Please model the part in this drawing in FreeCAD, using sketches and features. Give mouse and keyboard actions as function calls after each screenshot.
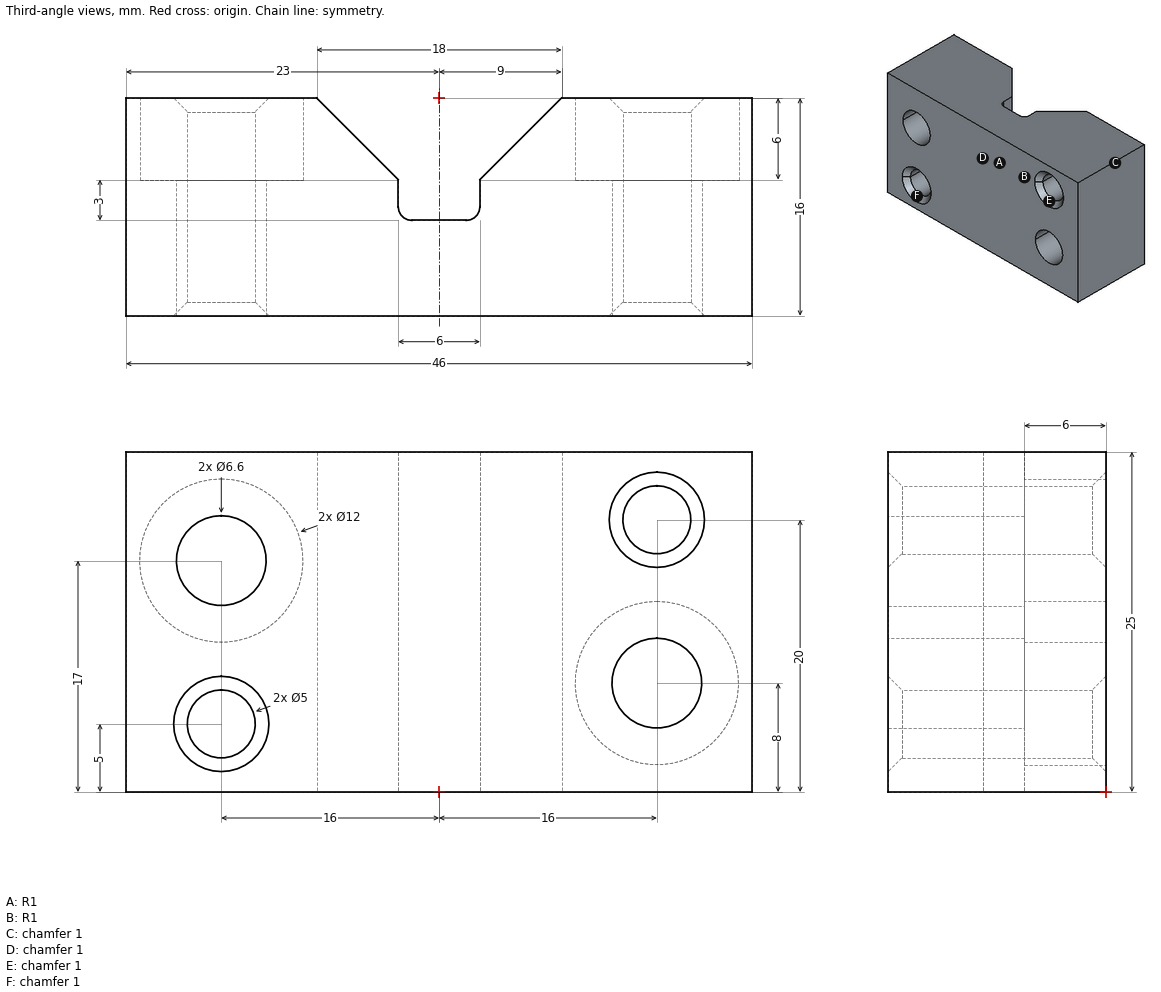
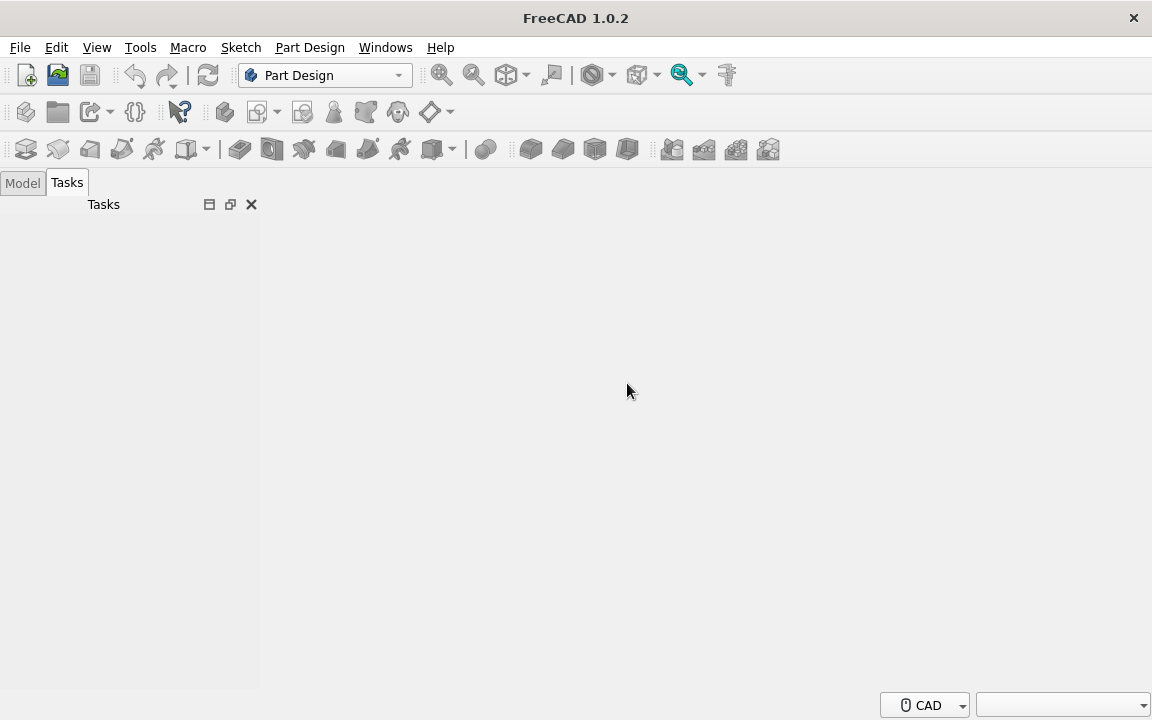
click(26, 76)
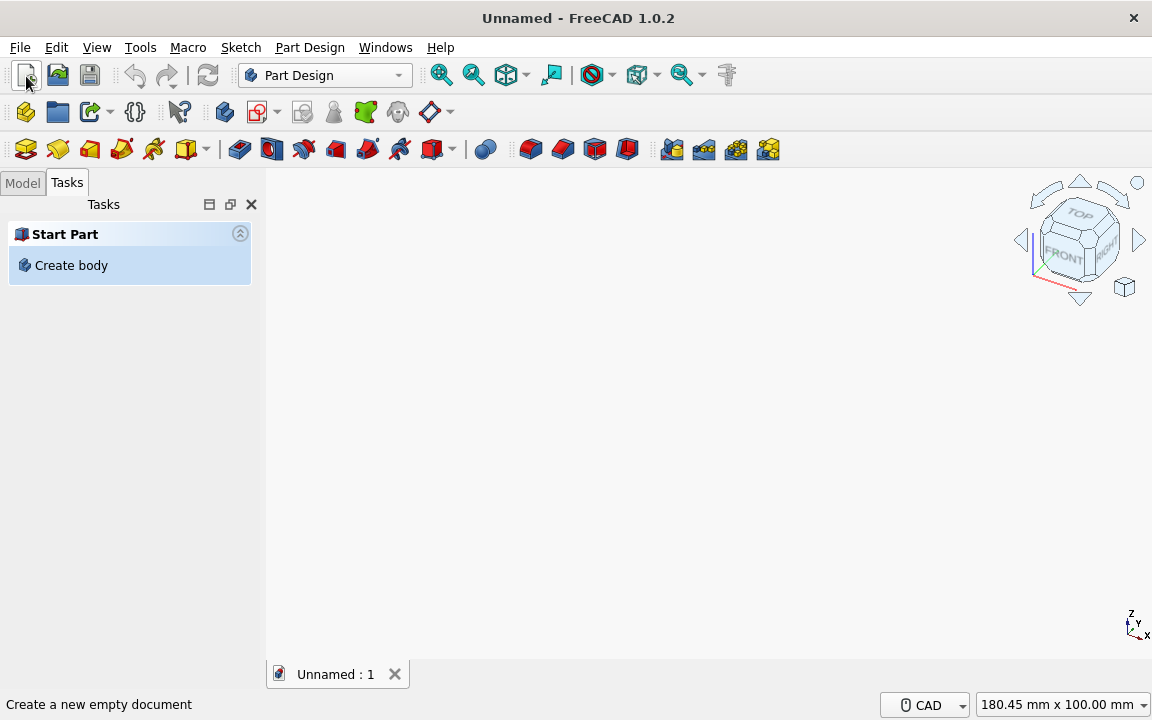
click(258, 112)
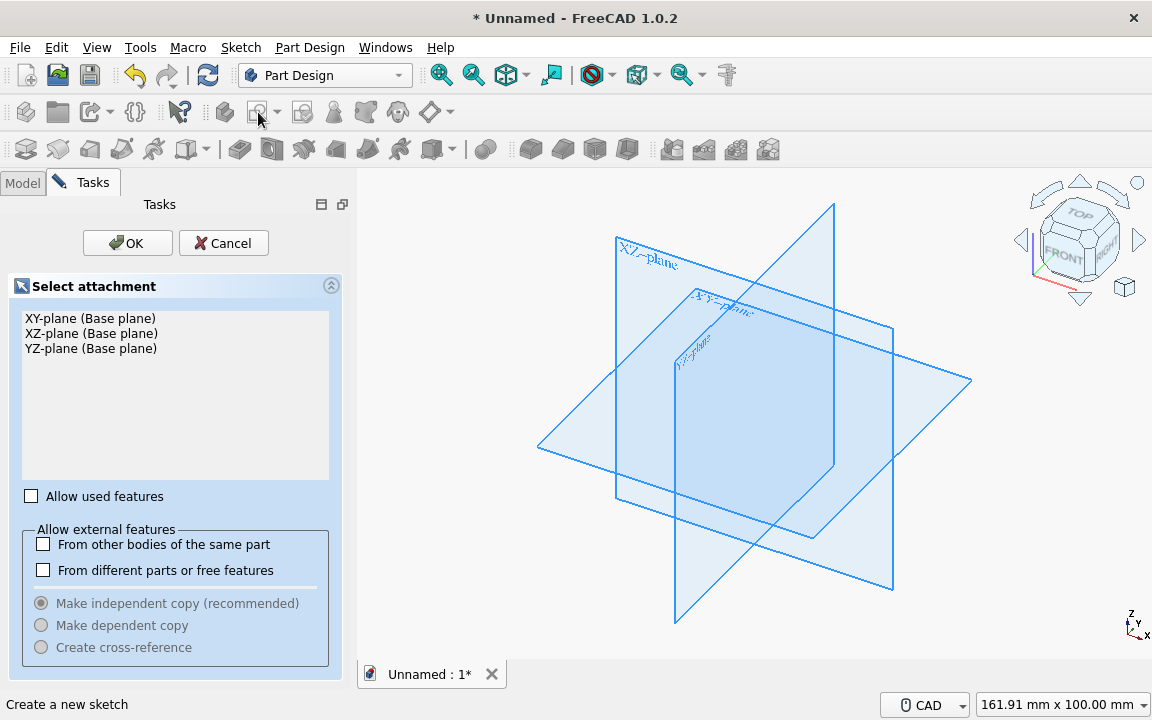
click(82, 318)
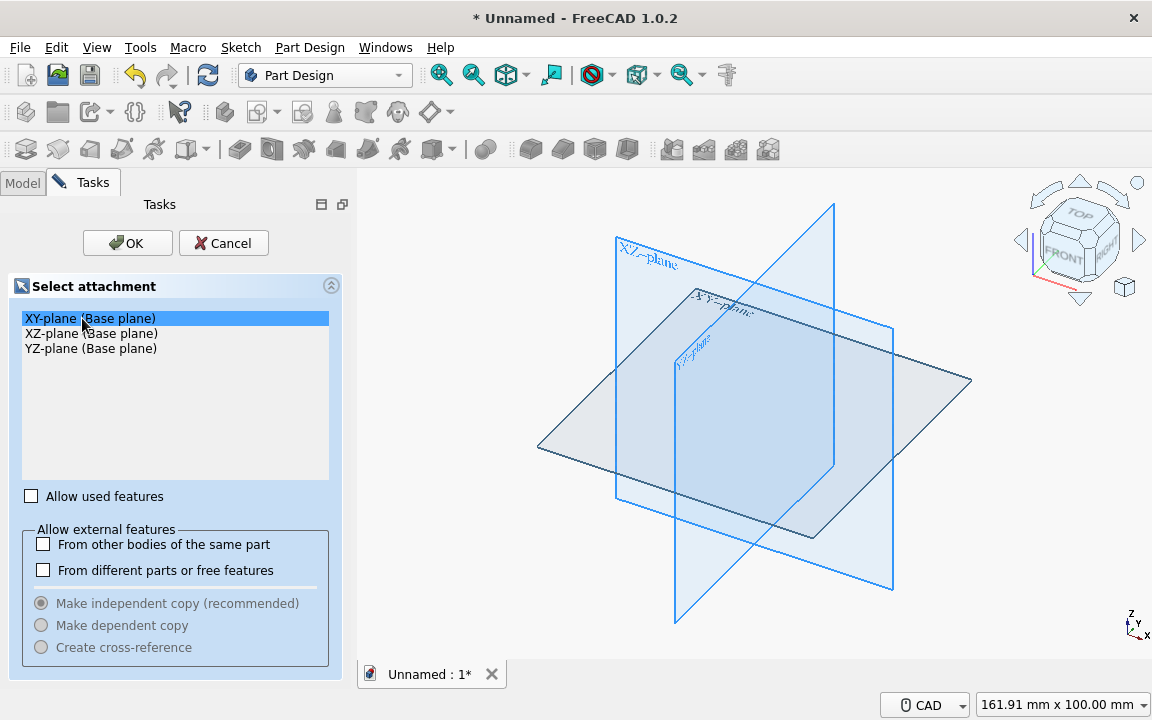
click(128, 243)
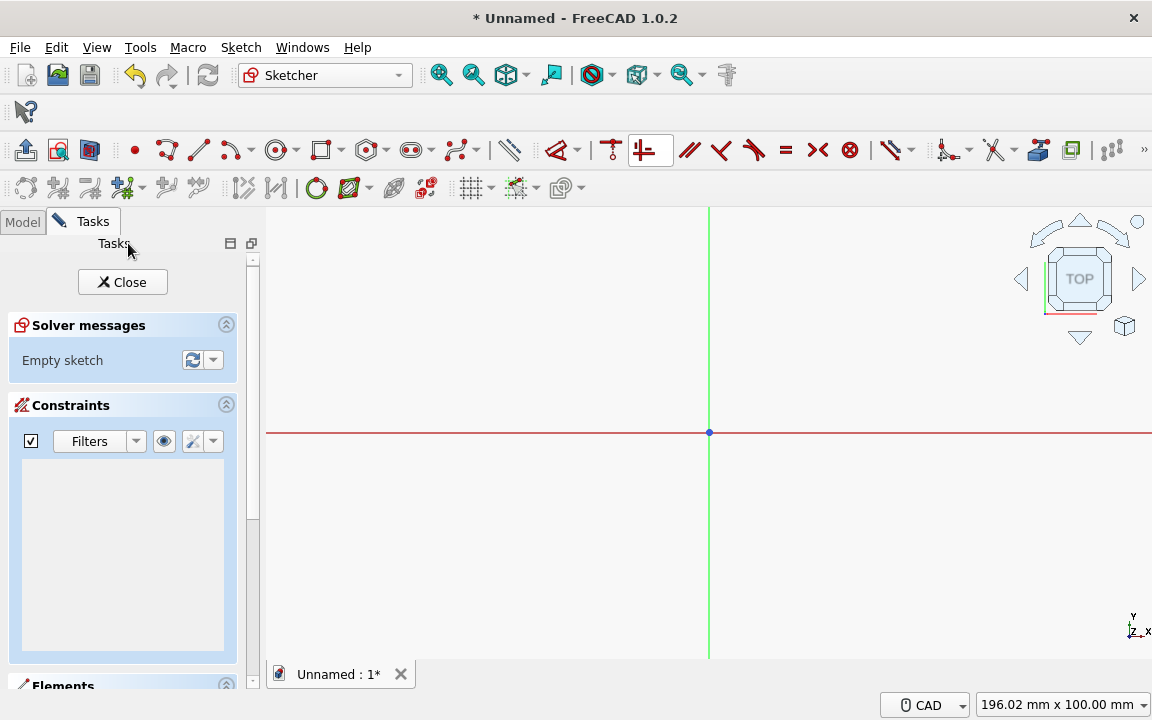
scroll(765, 499, up, 4)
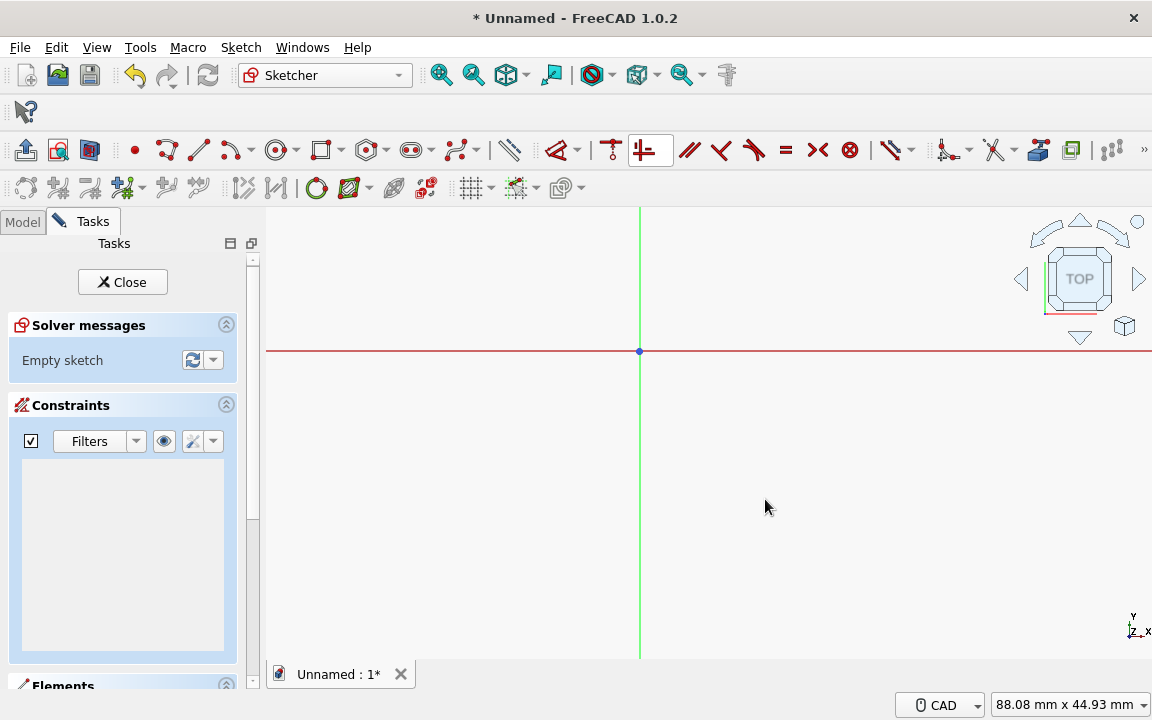
click(322, 150)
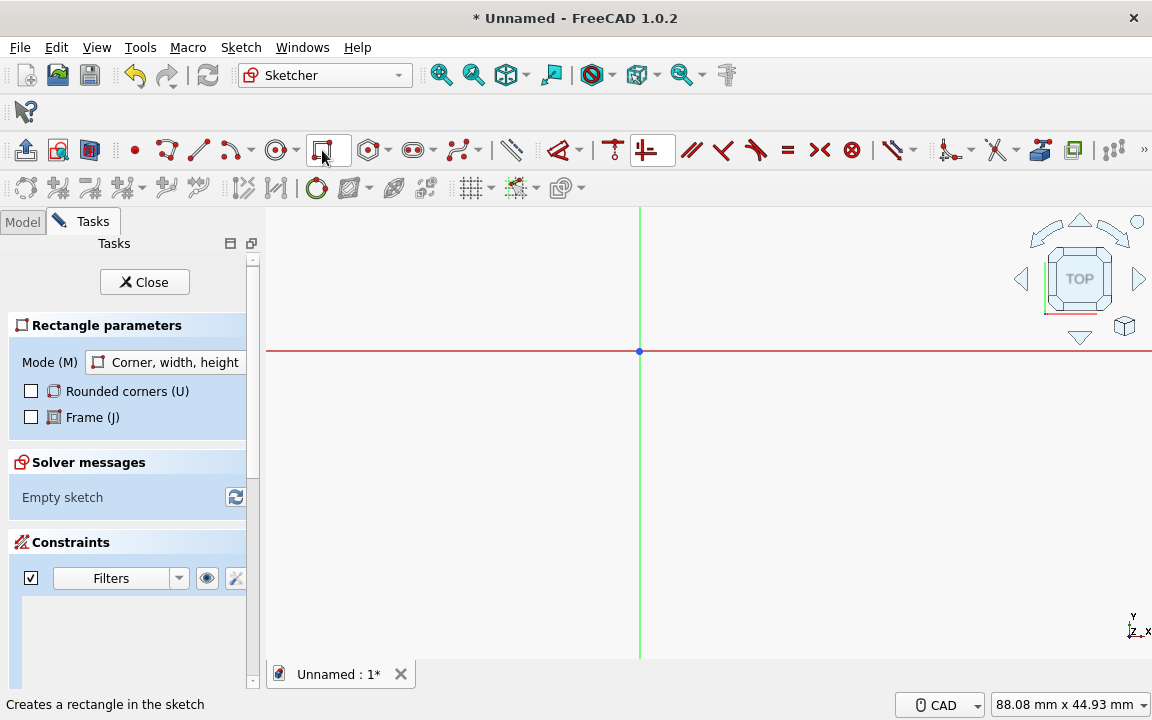
click(408, 351)
move(871, 512)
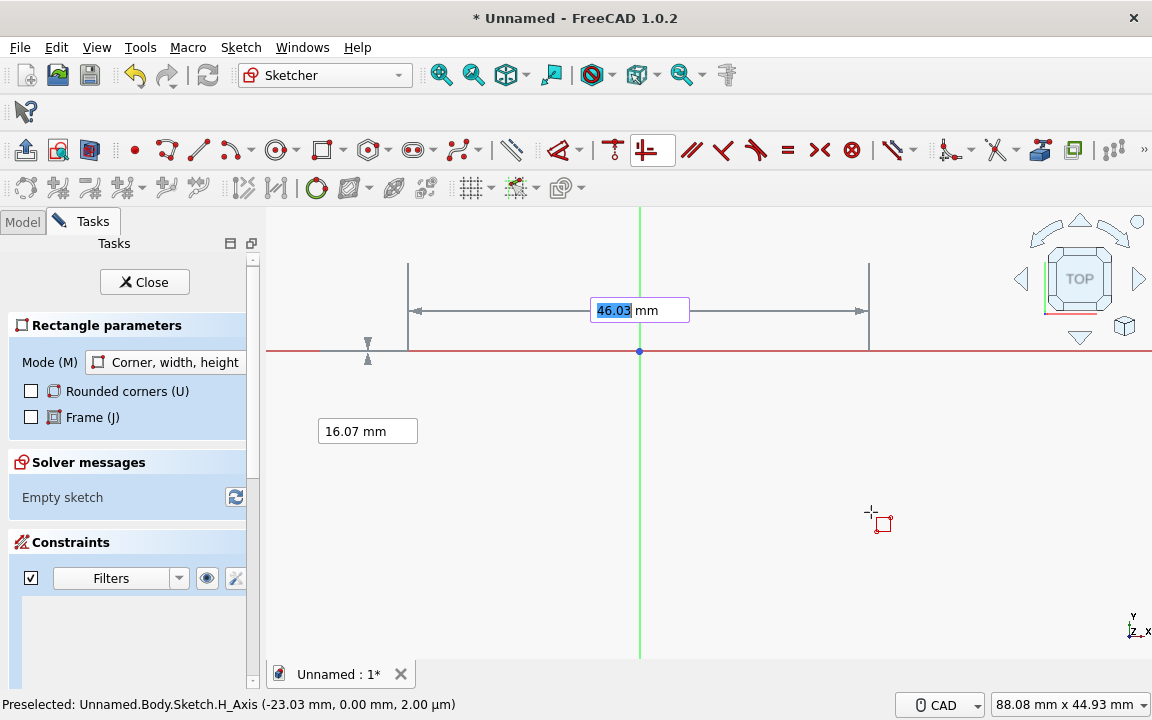
text(46)
key(Tab)
text(16)
key(Return)
key(Escape)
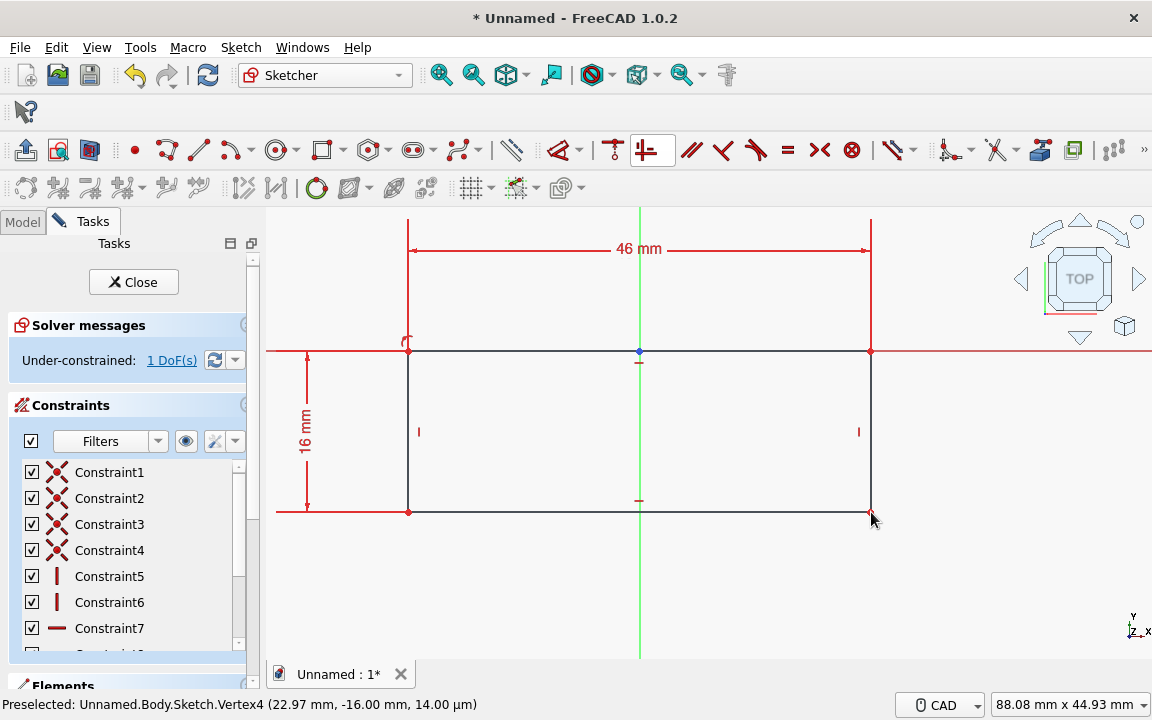
click(408, 351)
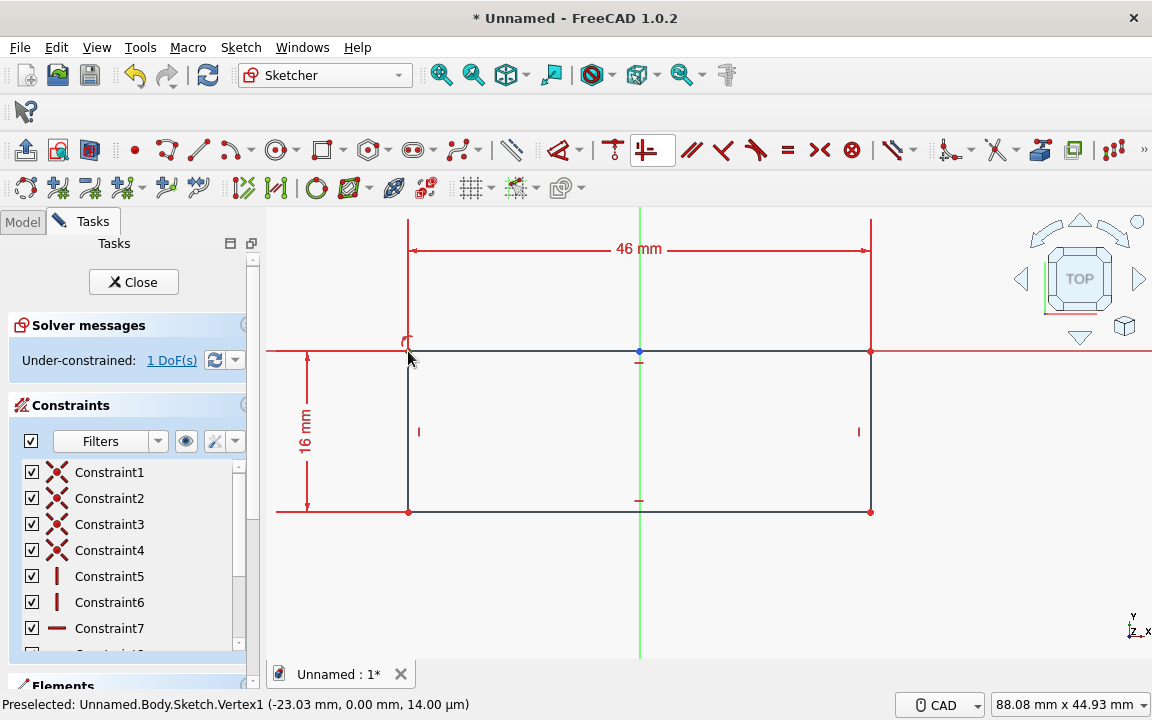
key(l)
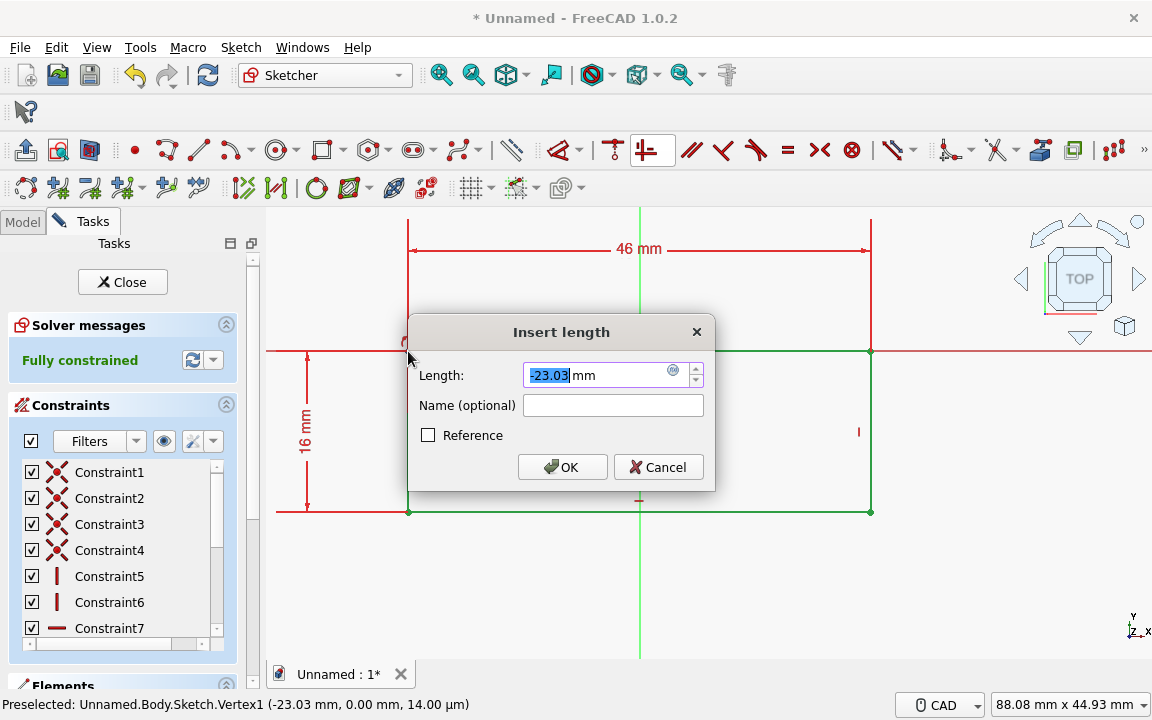
text(-23)
key(Return)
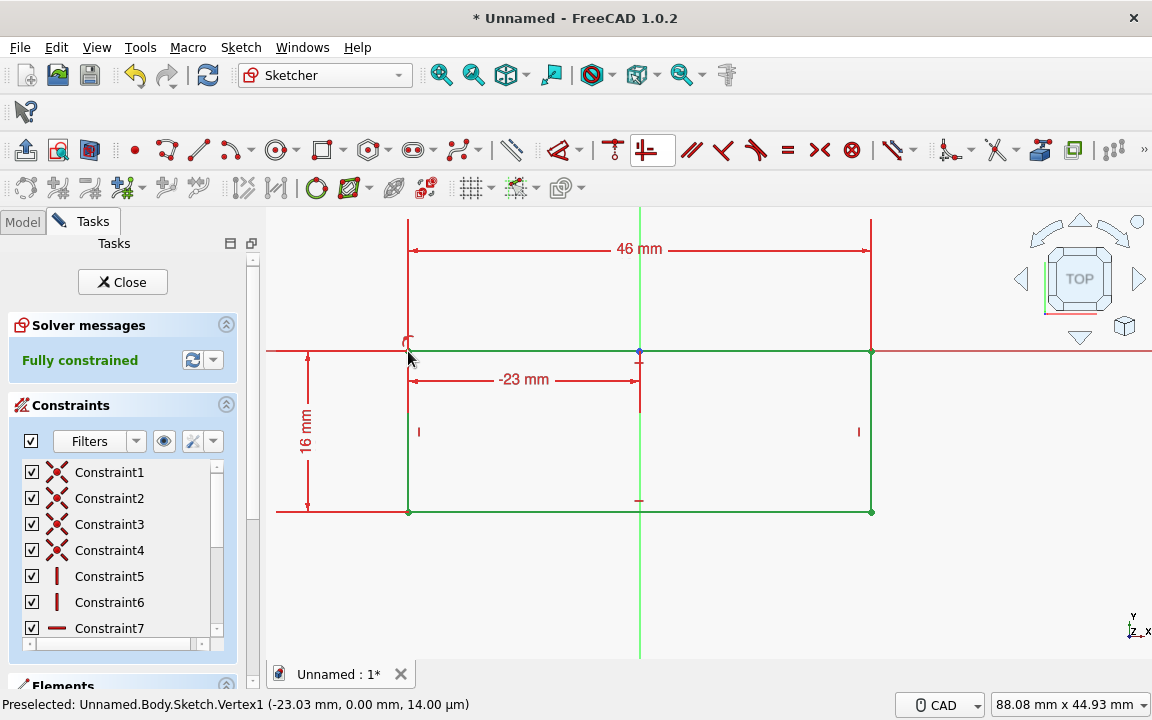
click(123, 282)